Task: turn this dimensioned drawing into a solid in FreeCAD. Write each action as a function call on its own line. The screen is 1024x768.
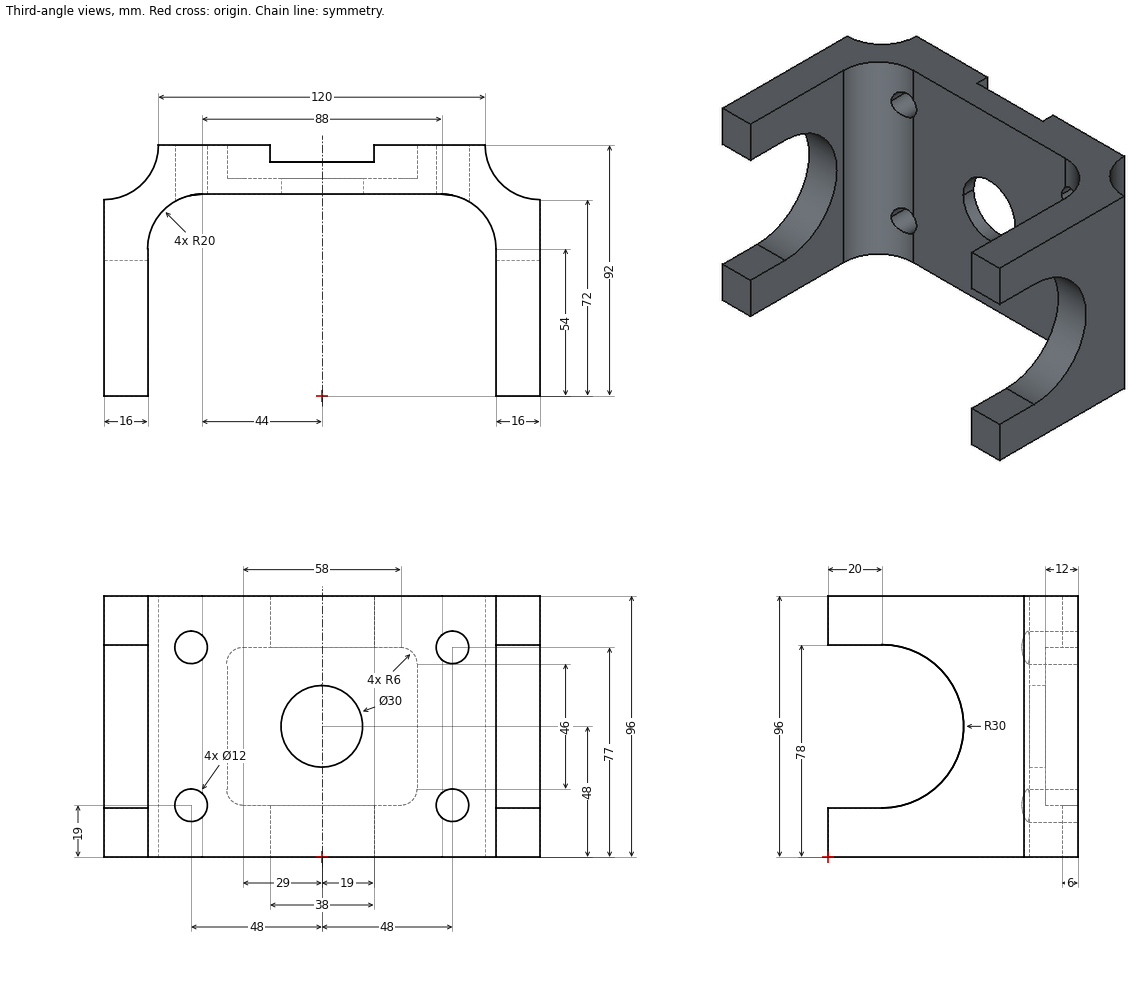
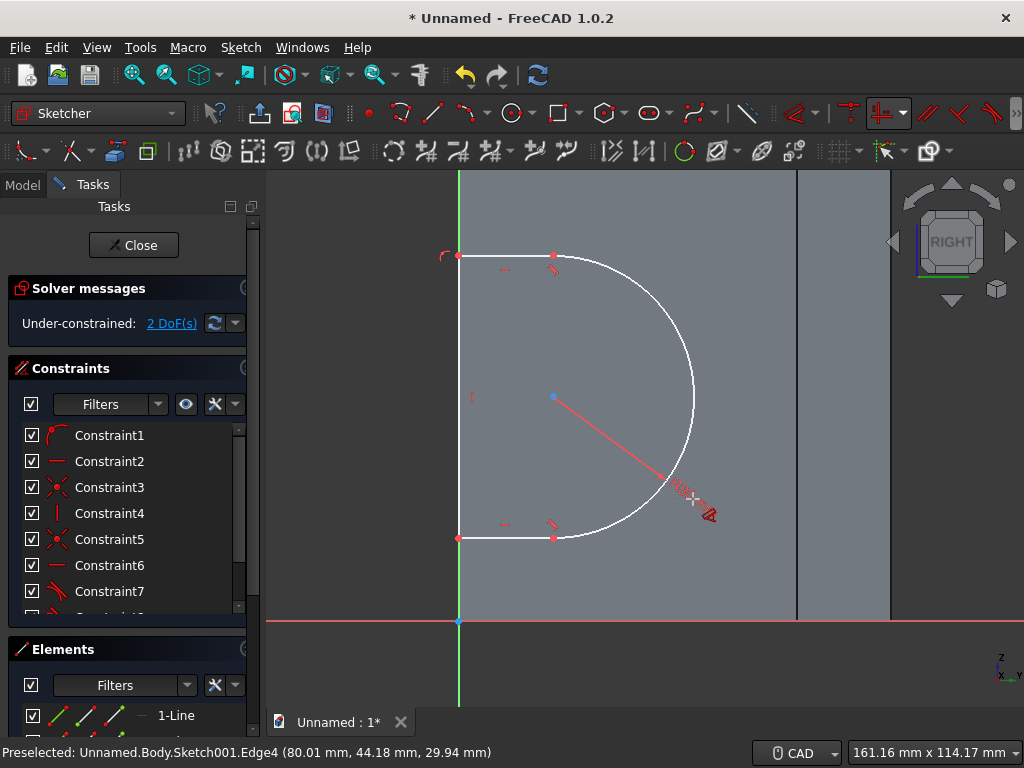
click(525, 256)
click(506, 222)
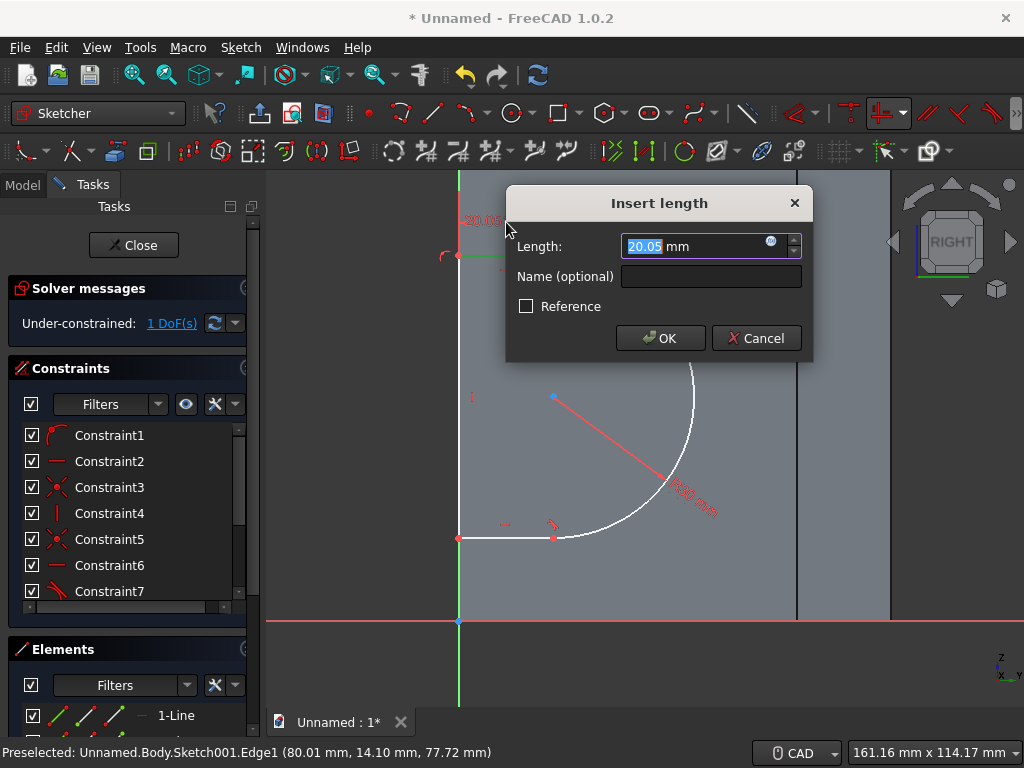
text(20)
key(Return)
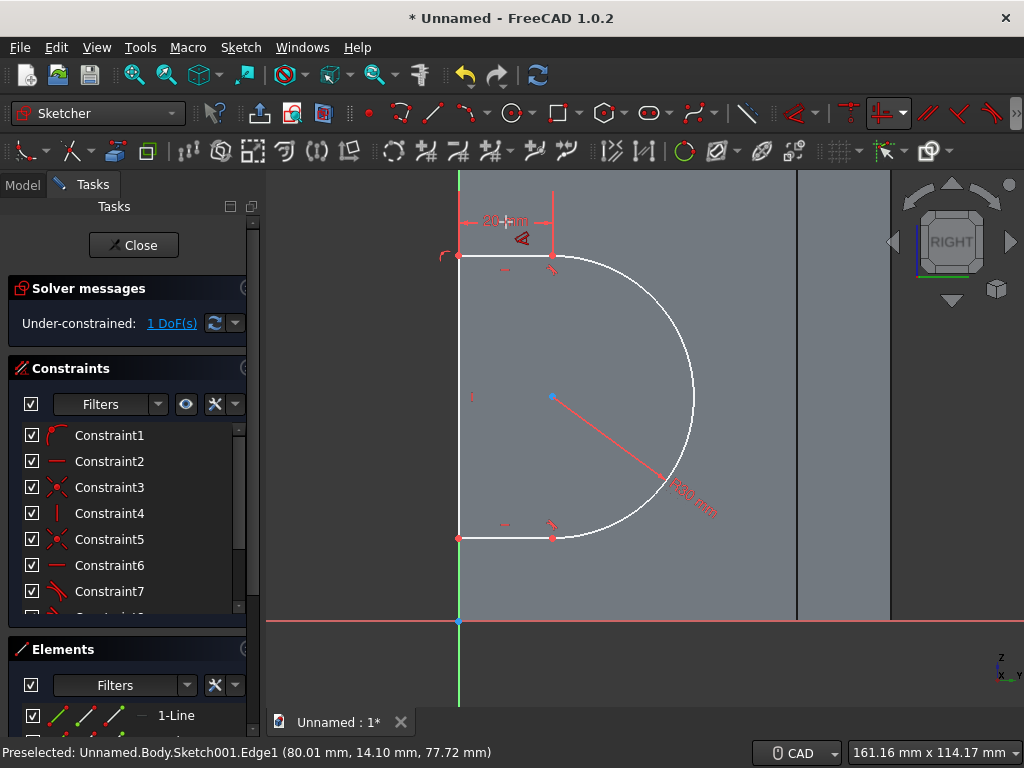
click(553, 256)
click(425, 439)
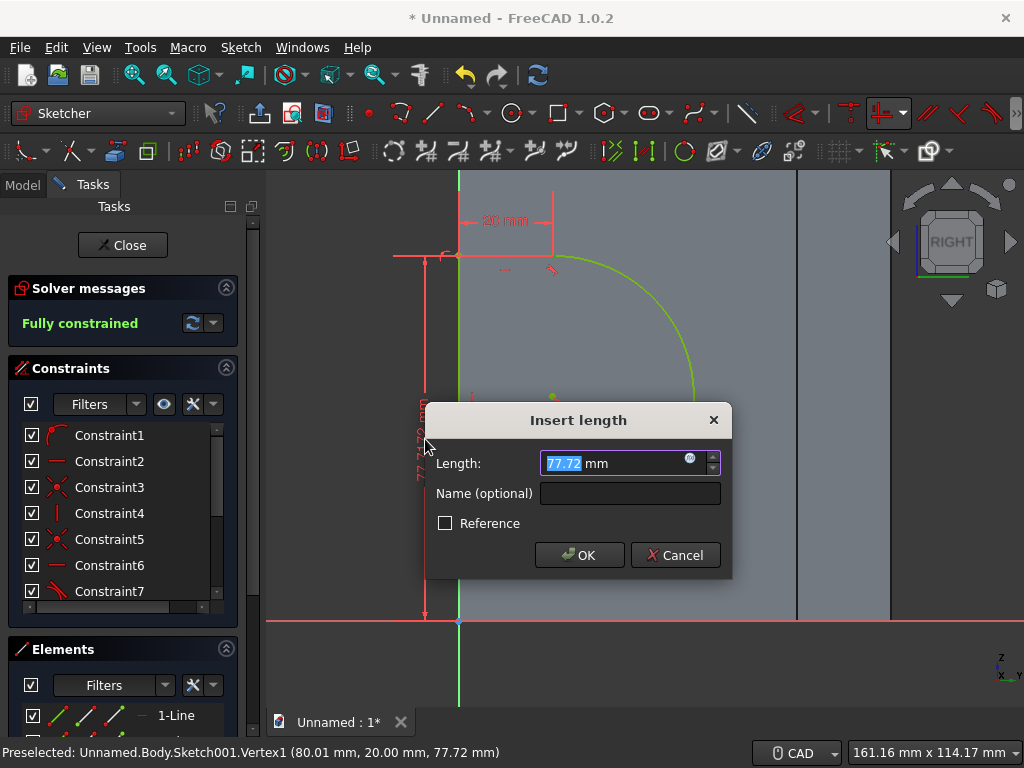
text(78)
key(Return)
key(Escape)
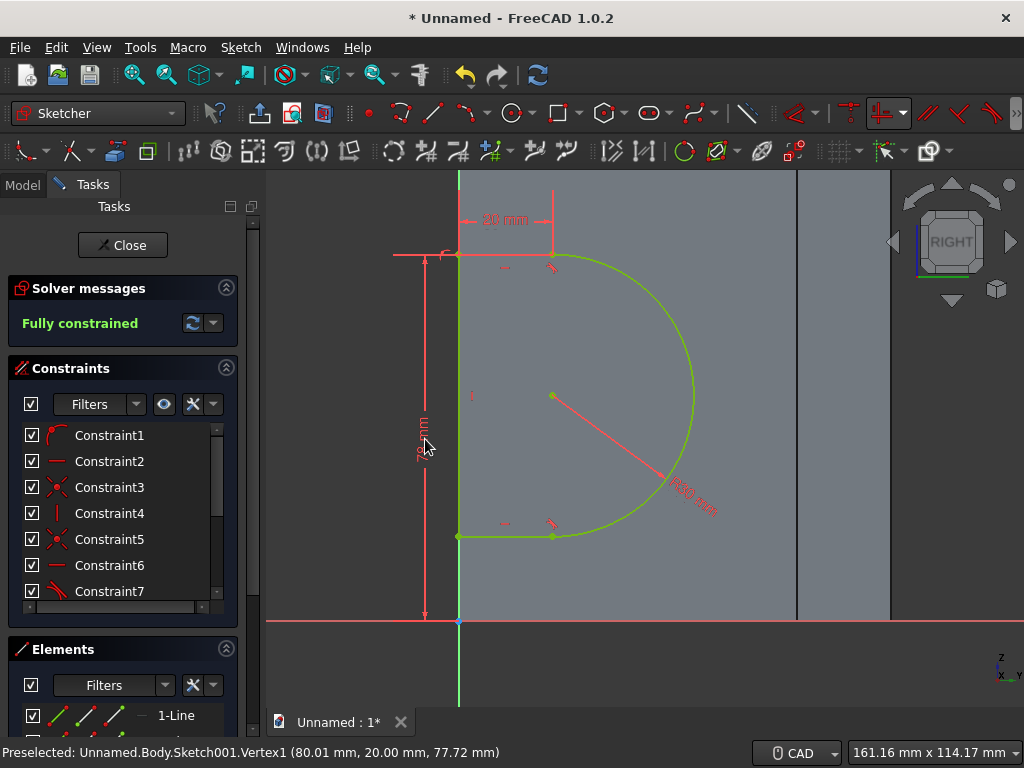
click(123, 245)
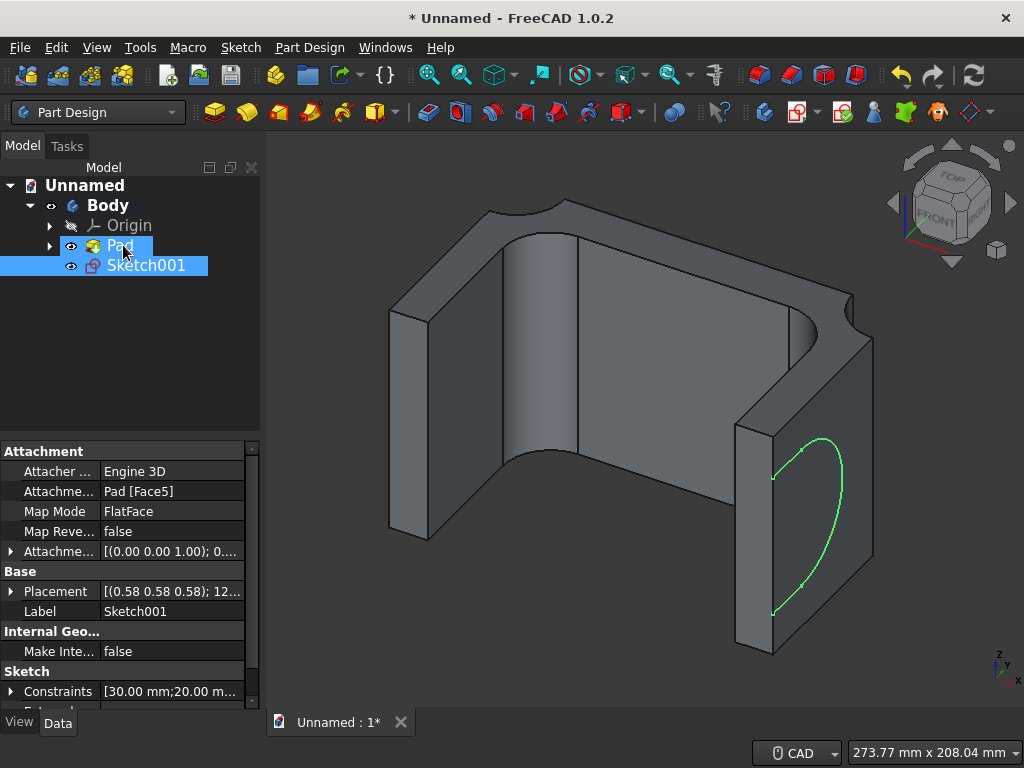
click(430, 112)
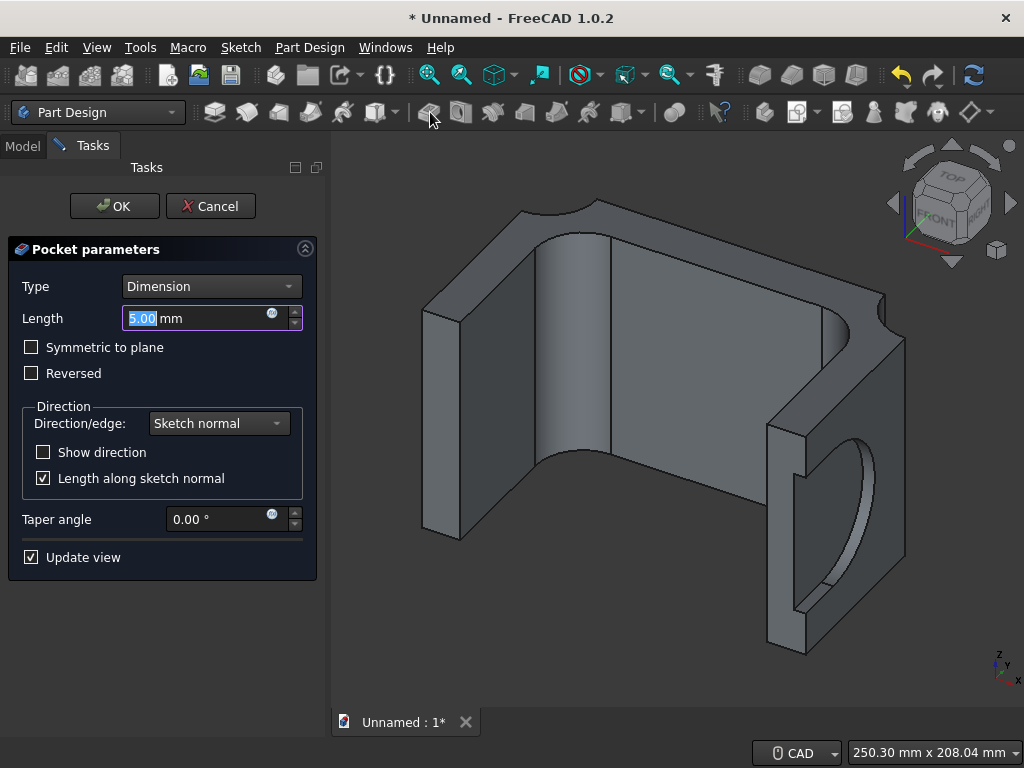
click(212, 286)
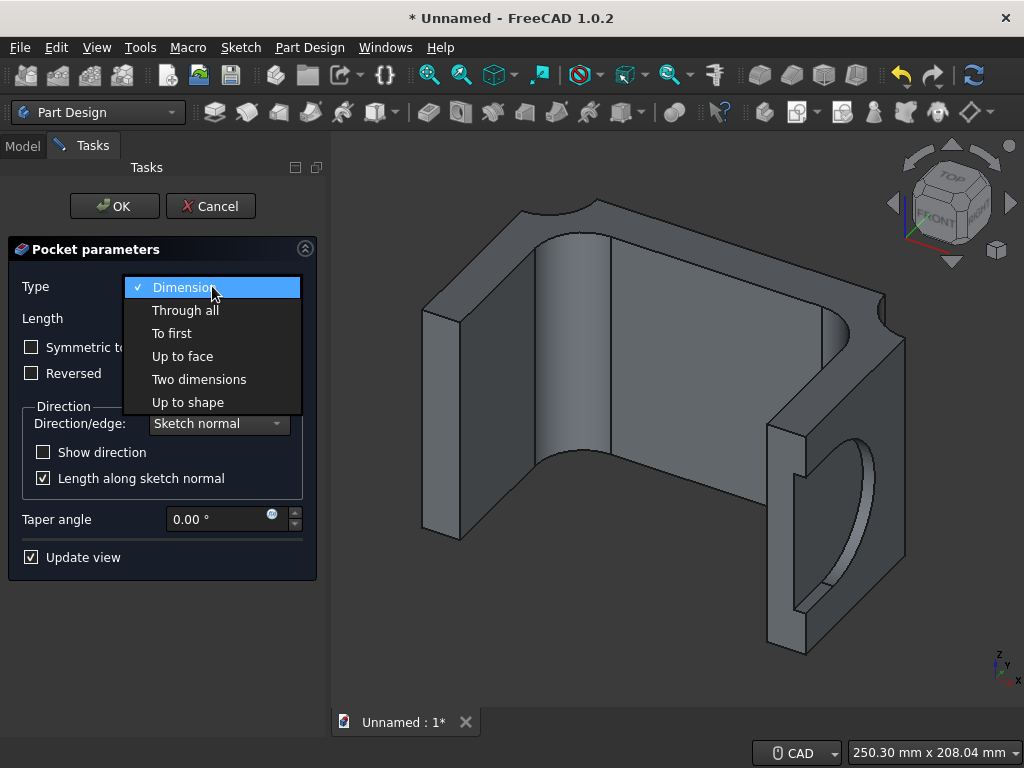
click(212, 310)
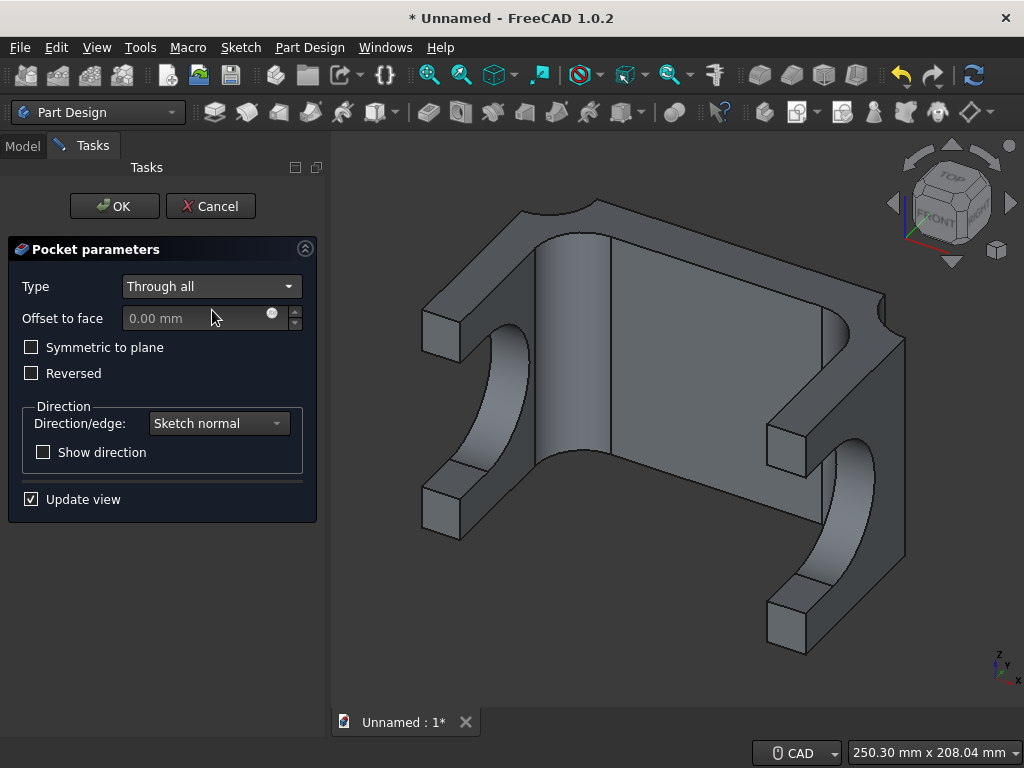
click(115, 206)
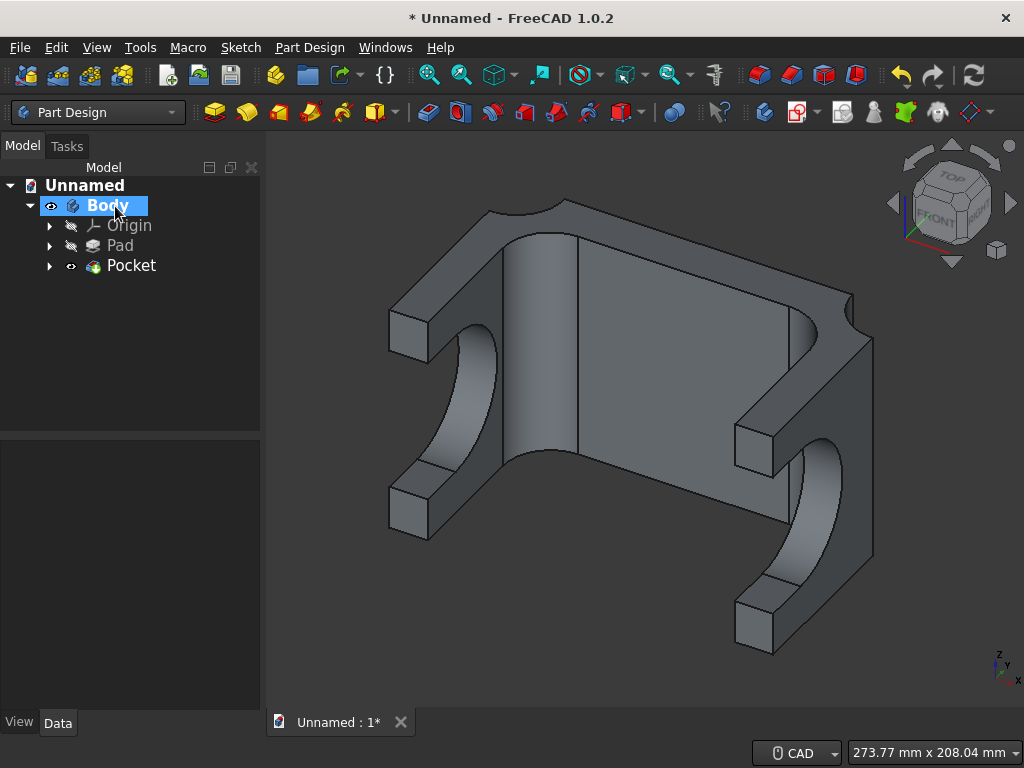
key(4)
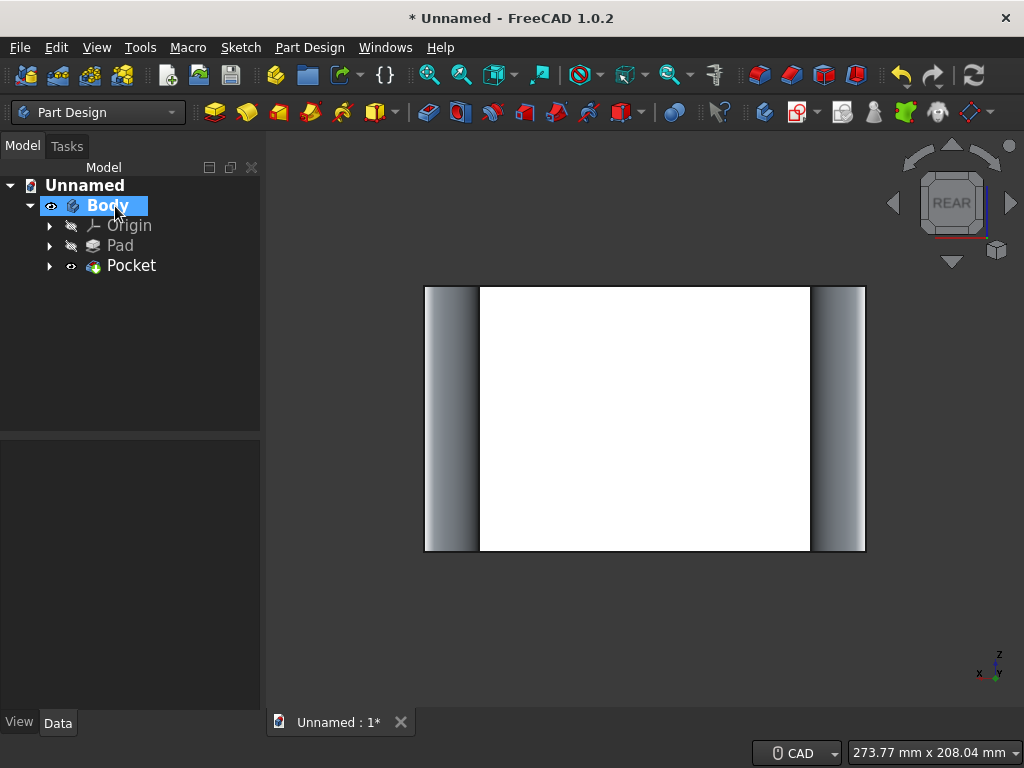
click(645, 418)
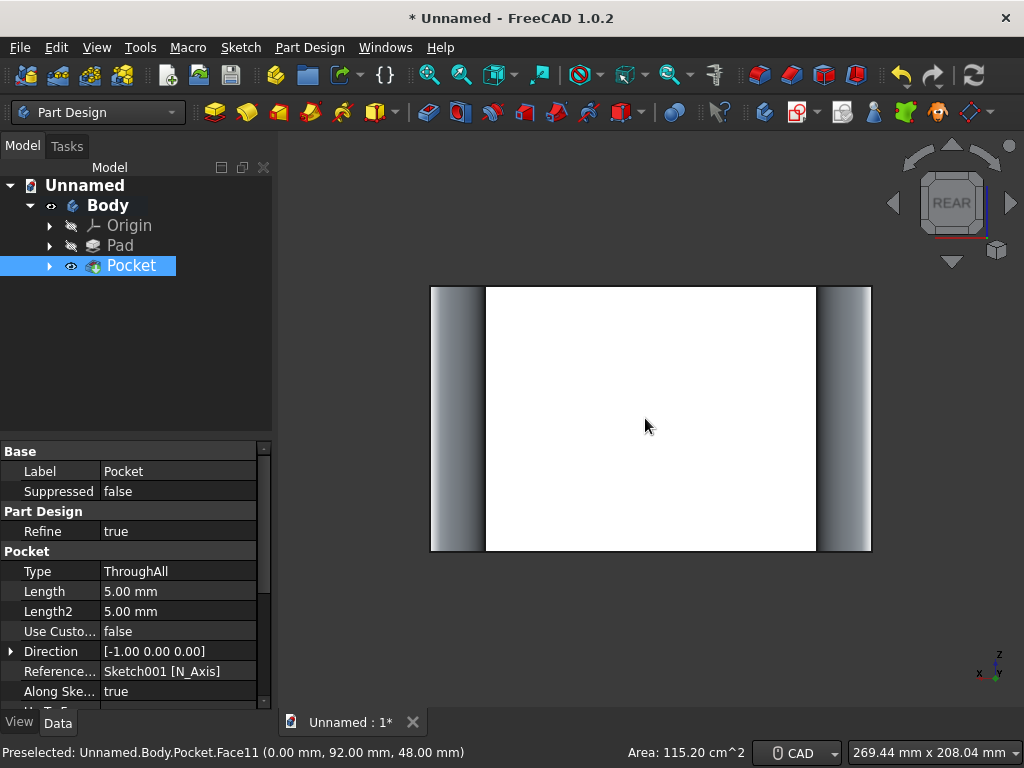
click(798, 112)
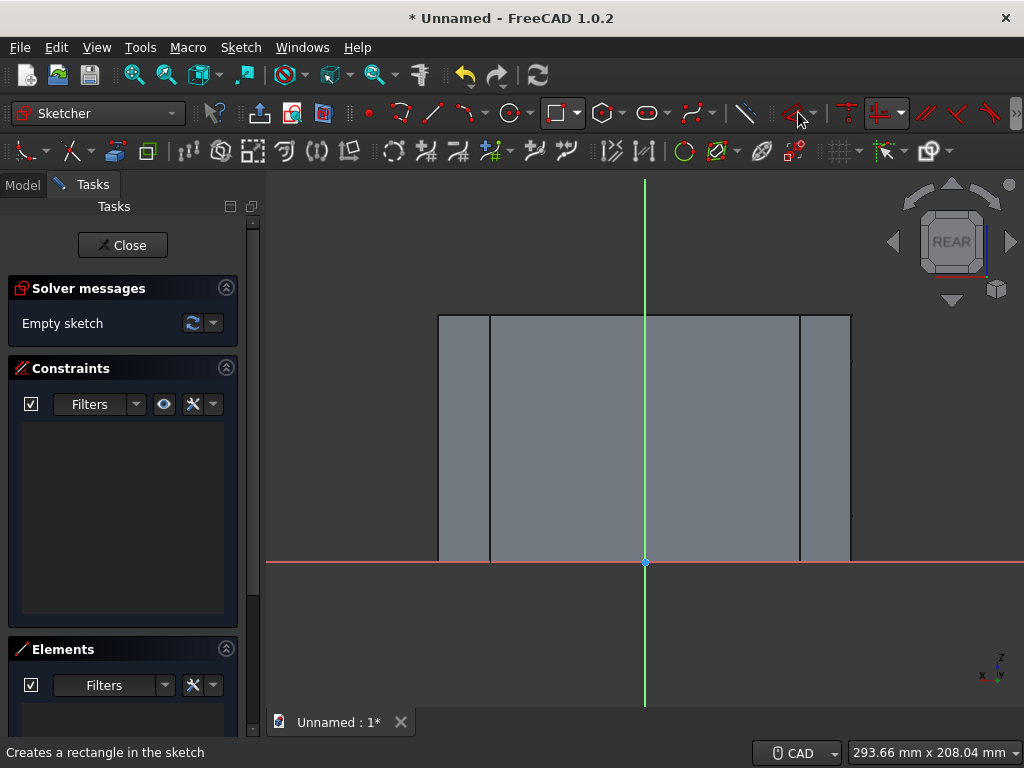
scroll(784, 439, up, 2)